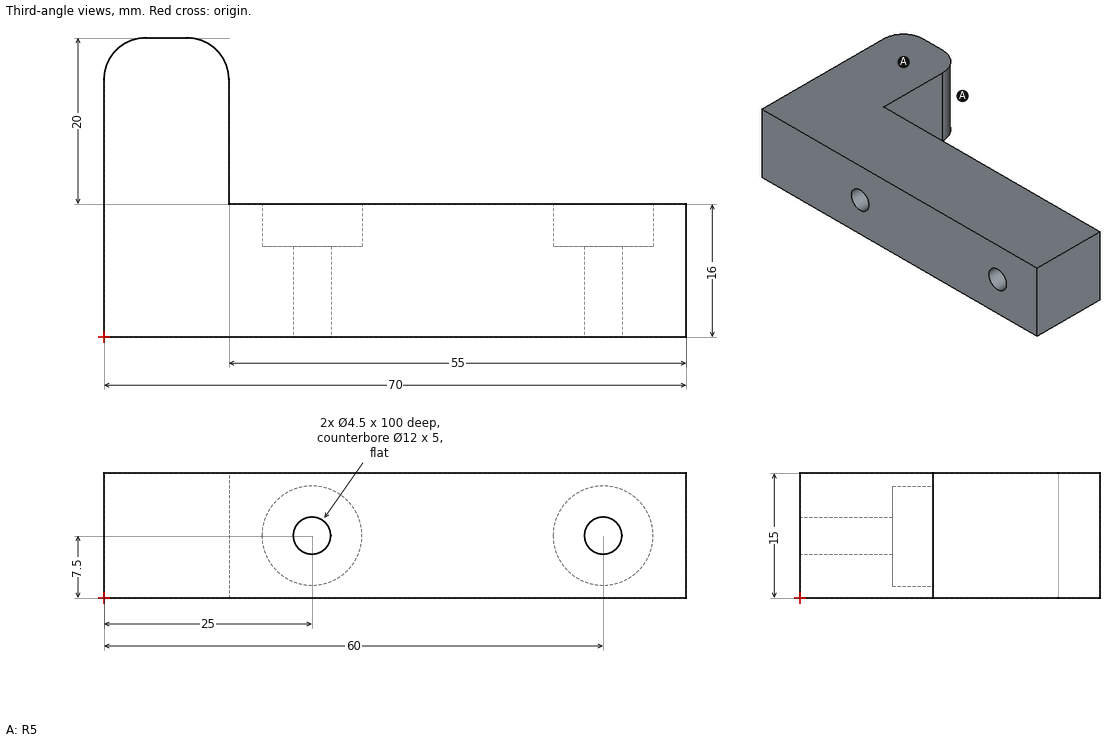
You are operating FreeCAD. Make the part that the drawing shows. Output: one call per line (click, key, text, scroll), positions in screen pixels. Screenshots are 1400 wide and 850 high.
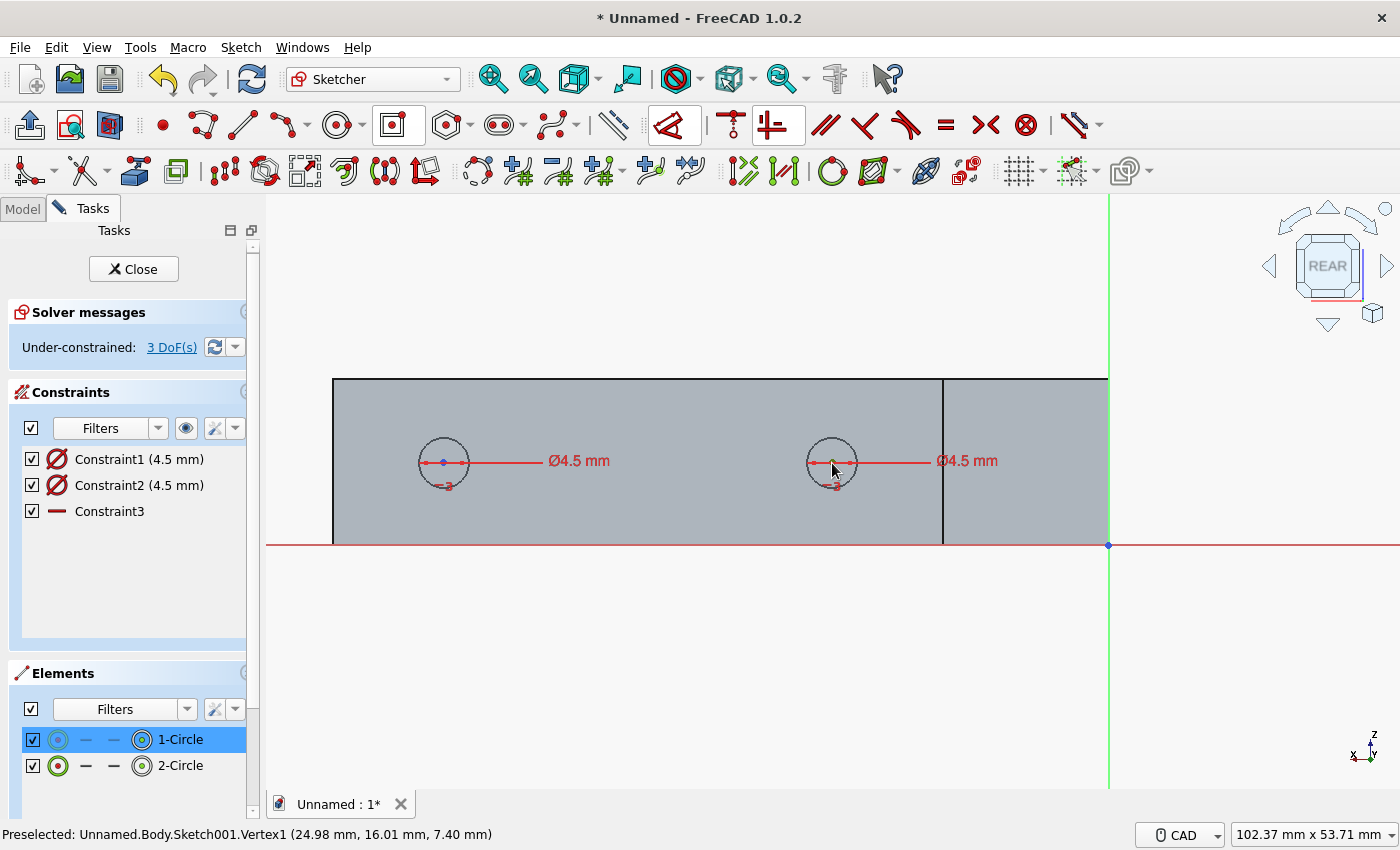
click(696, 126)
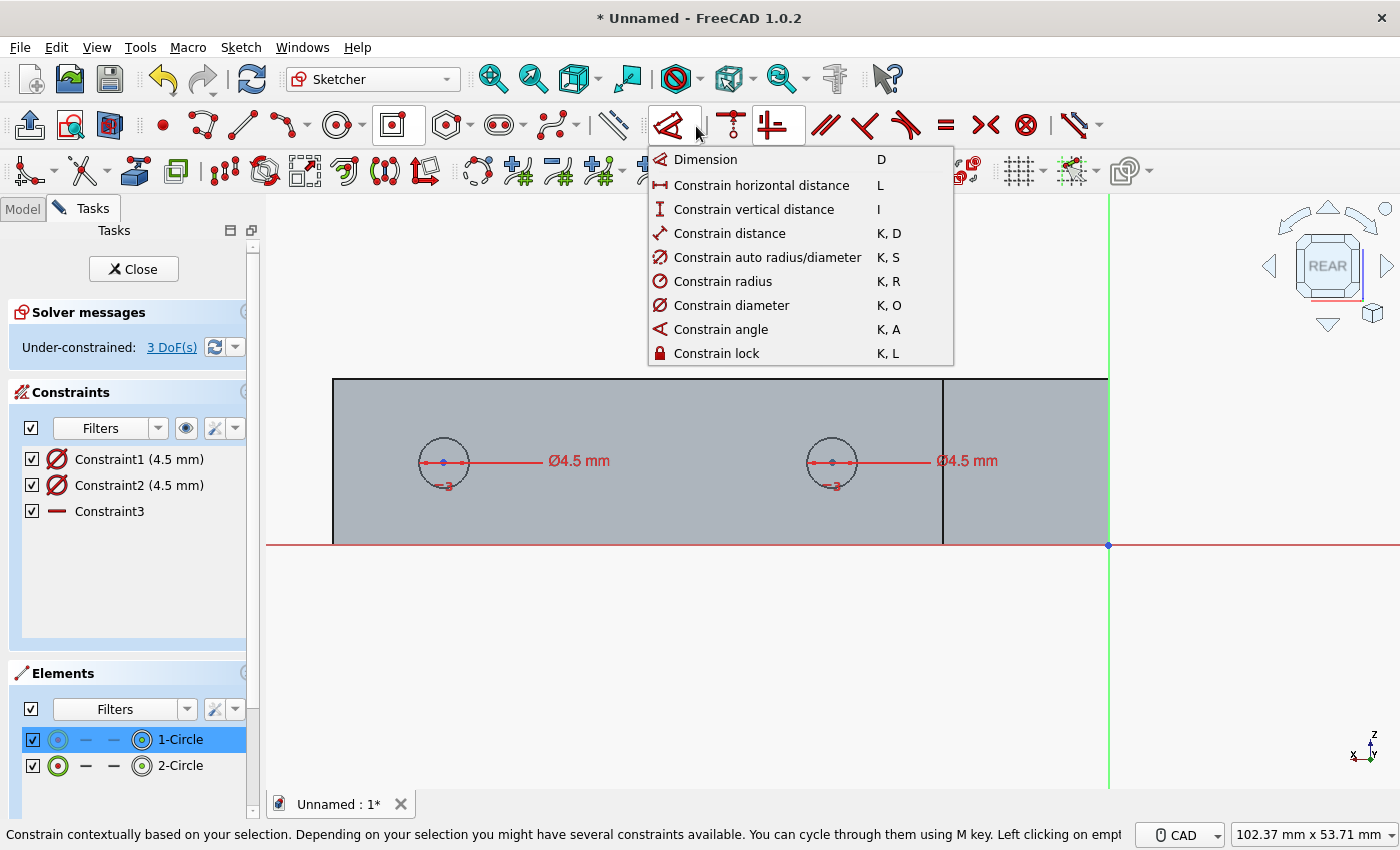
click(801, 185)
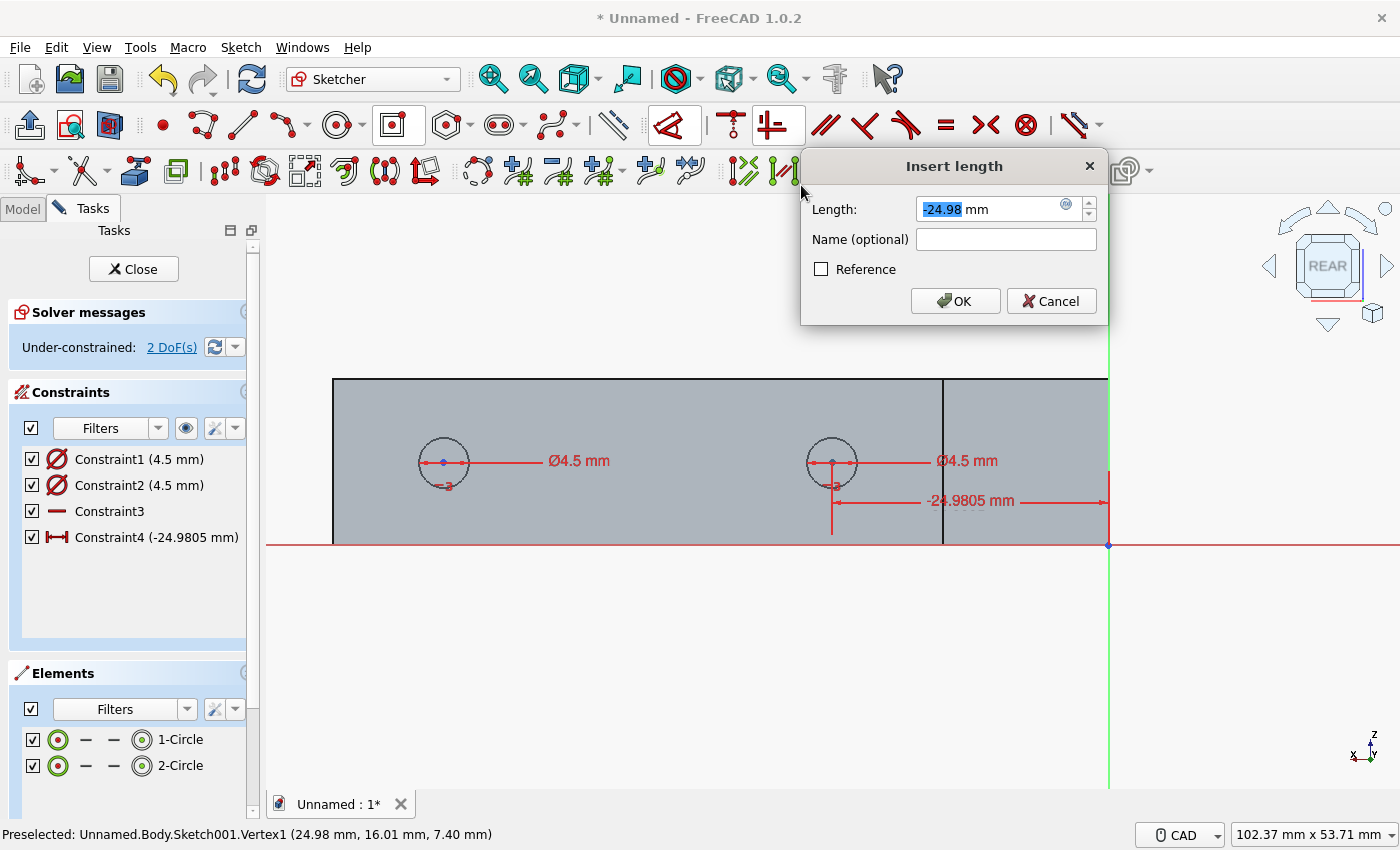
text(-25)
key(Return)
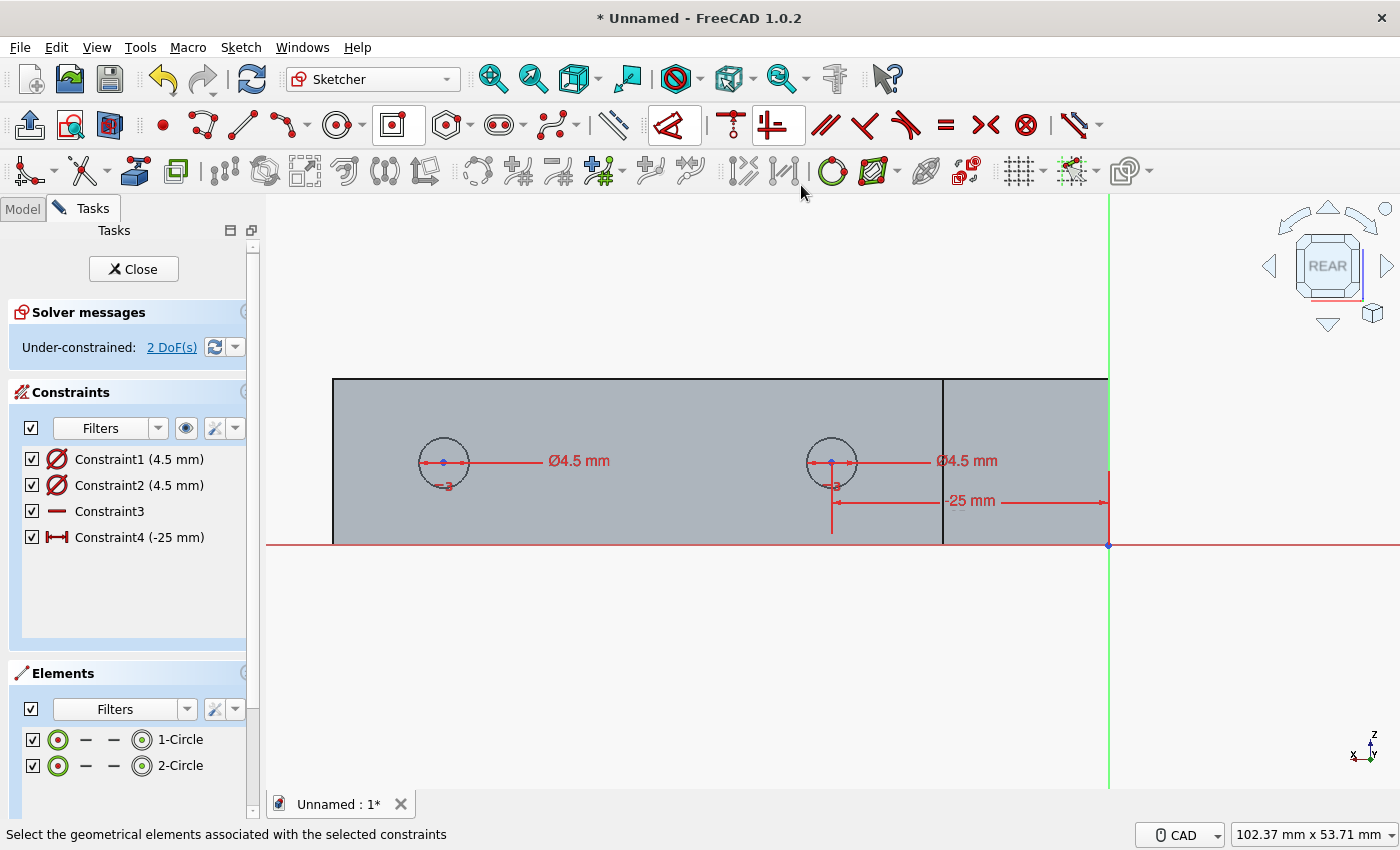
click(444, 463)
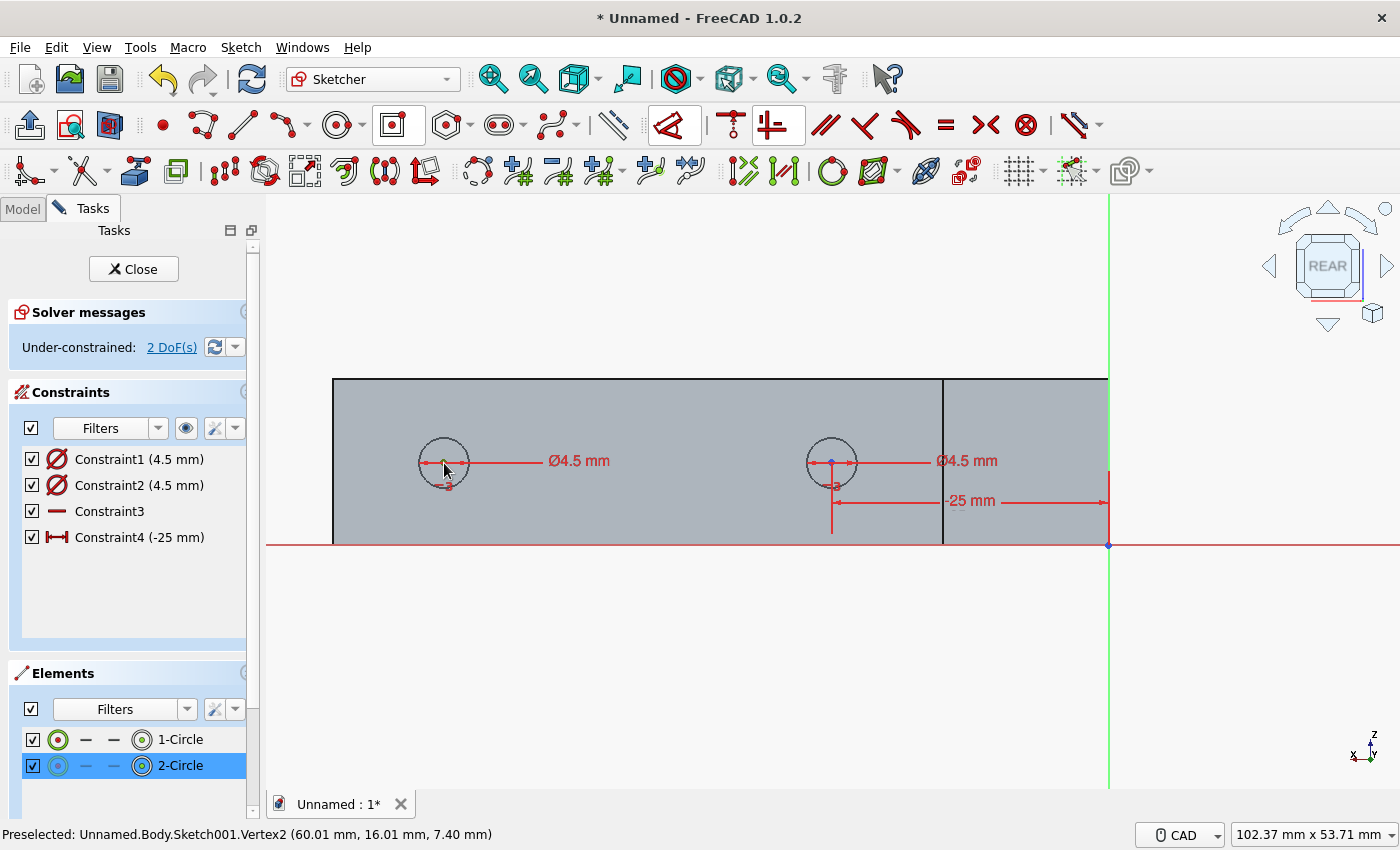
click(696, 126)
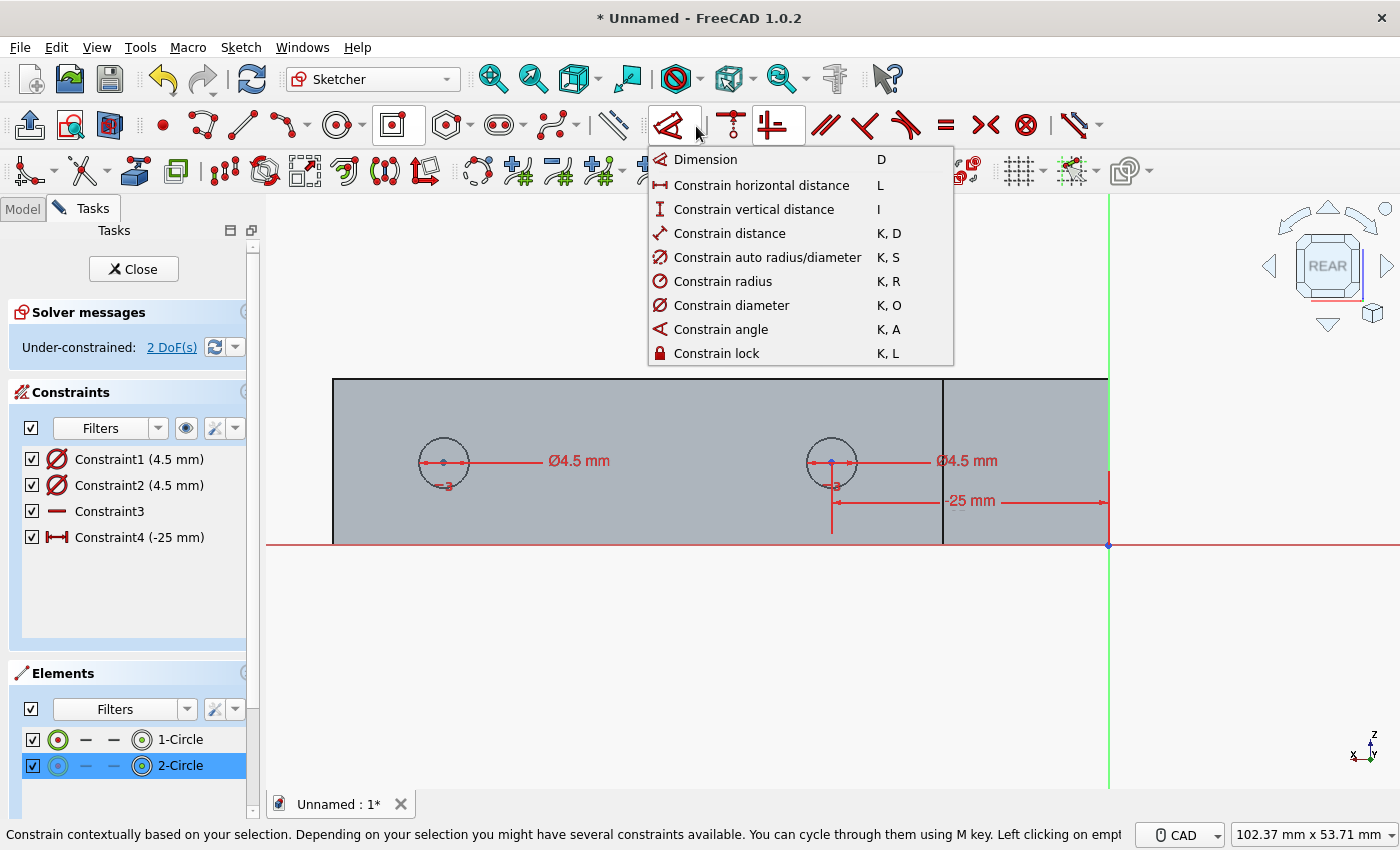
click(801, 185)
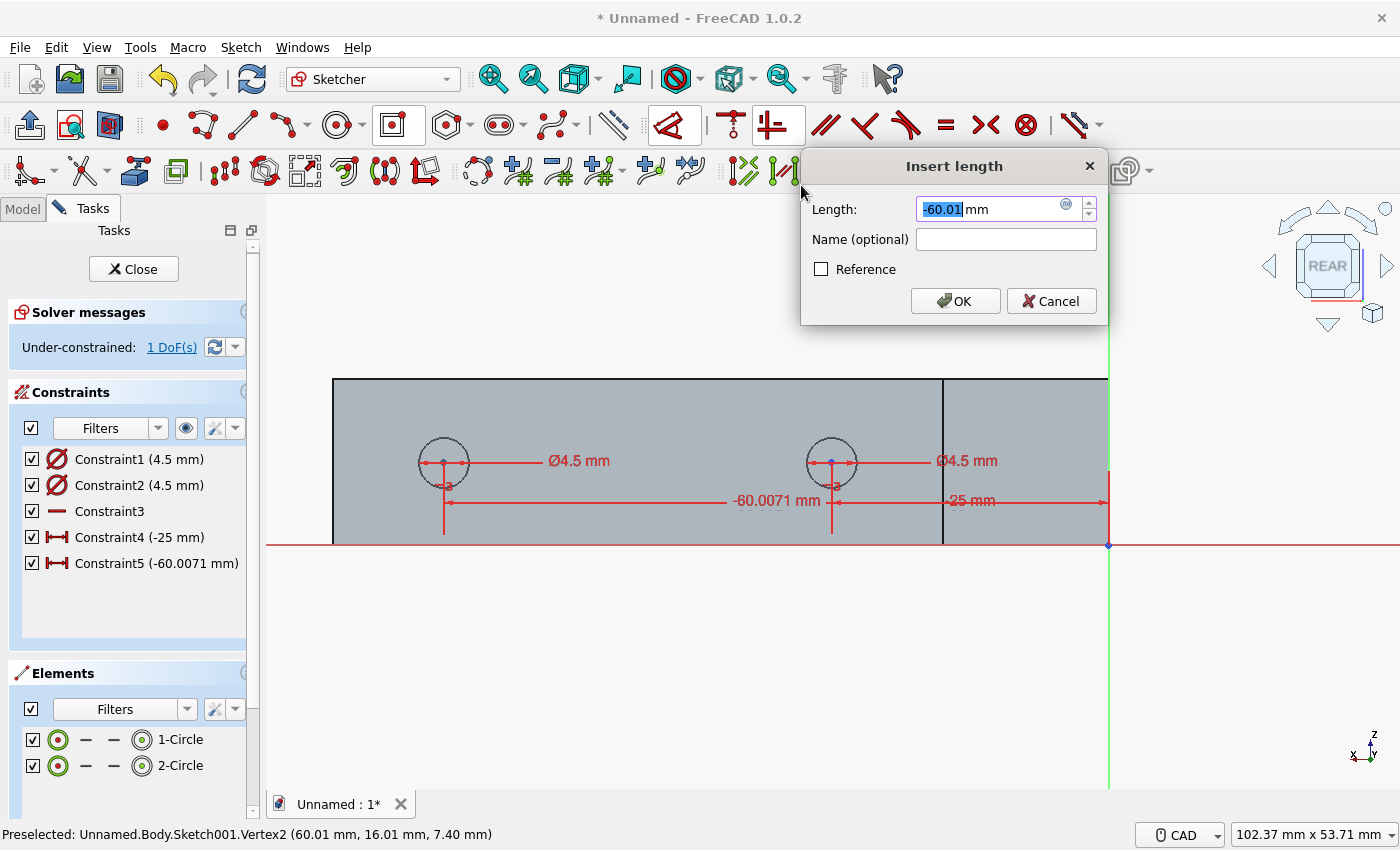
text(-60)
key(Return)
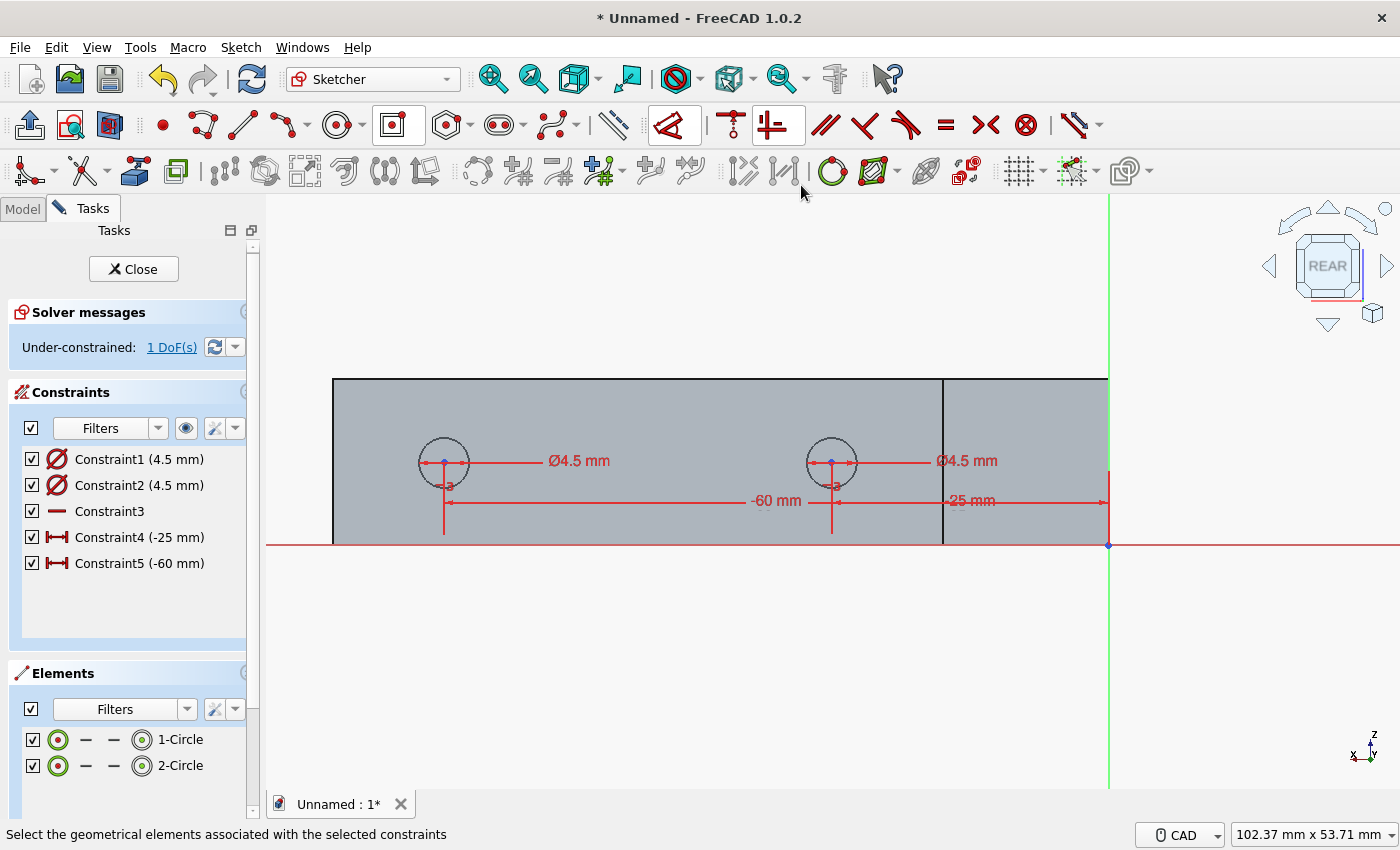
click(832, 463)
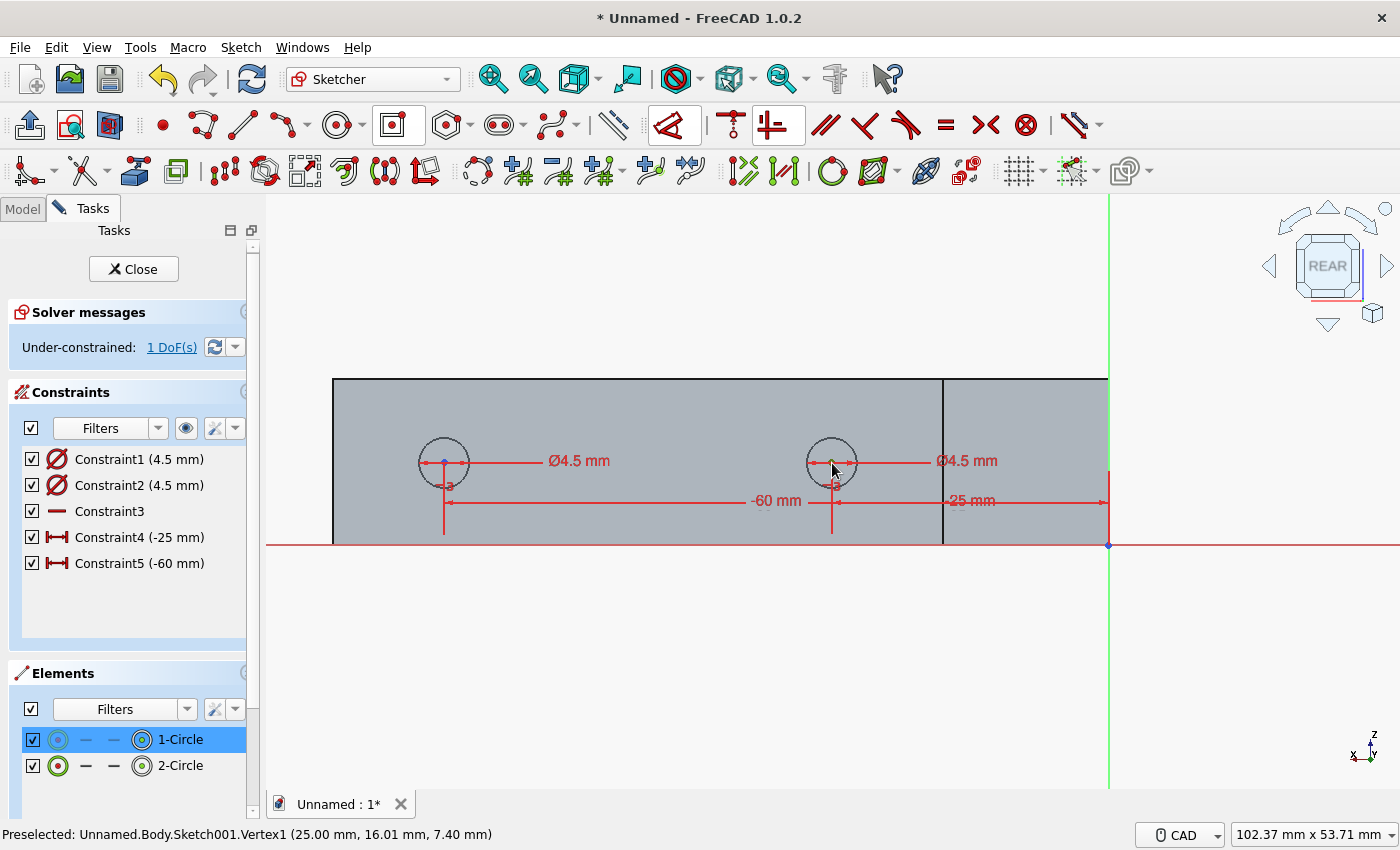
click(696, 126)